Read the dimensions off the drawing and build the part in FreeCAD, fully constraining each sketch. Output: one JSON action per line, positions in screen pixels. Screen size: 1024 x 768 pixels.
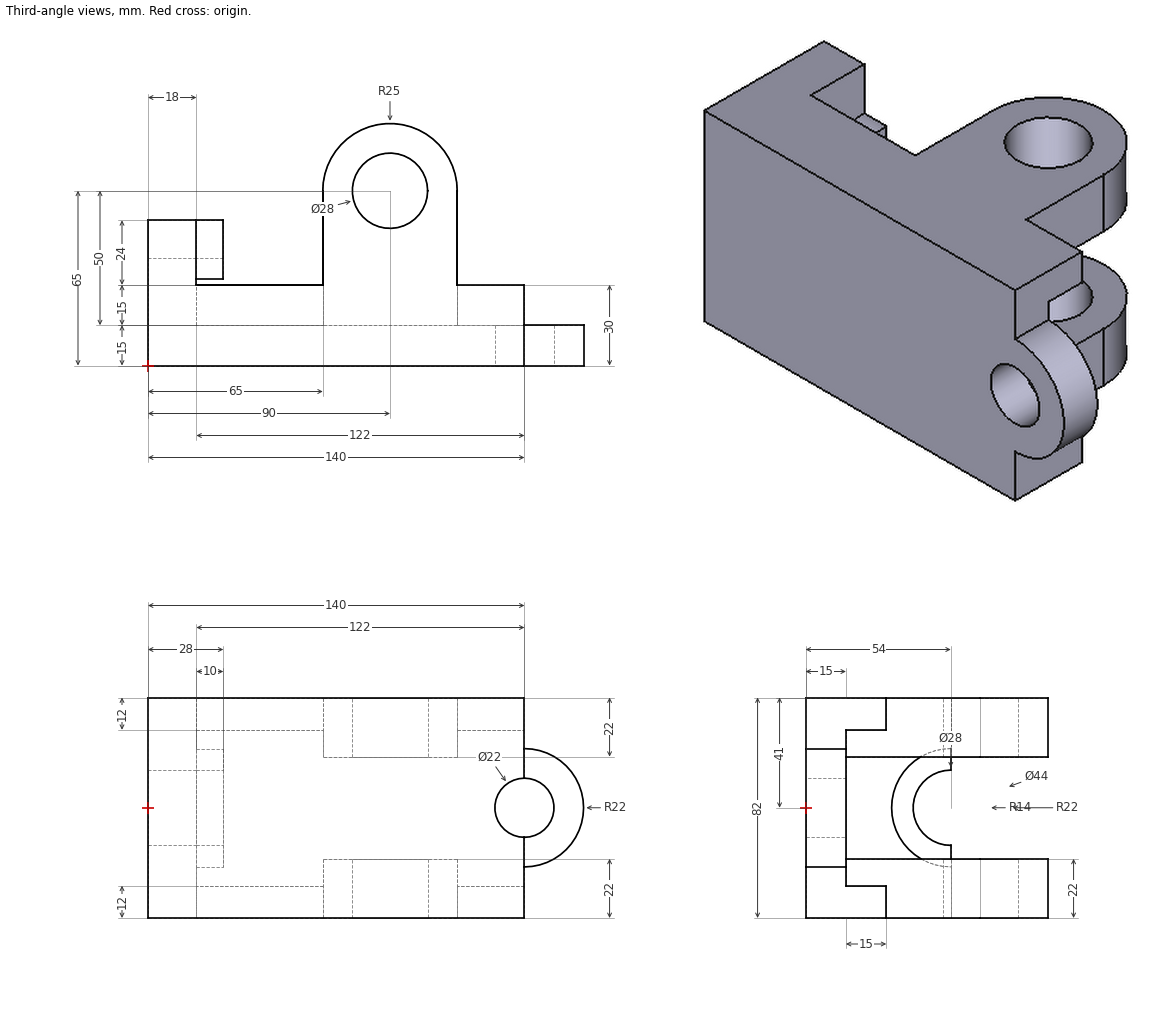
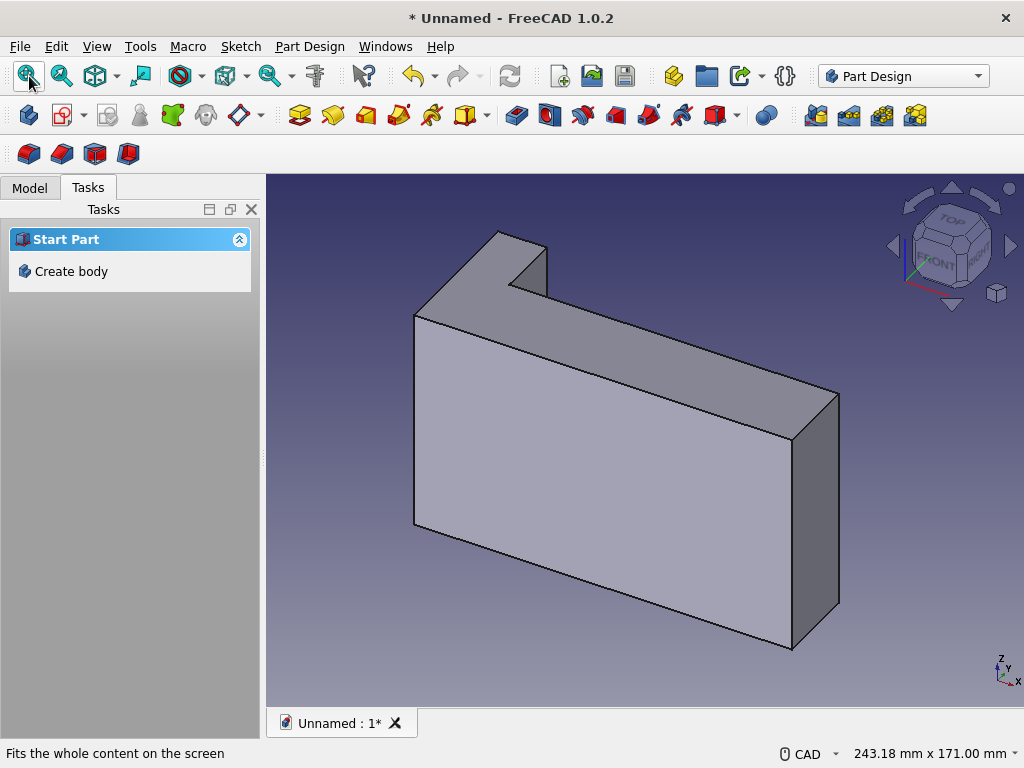
{"action": "left_click", "coordinate": [815, 461]}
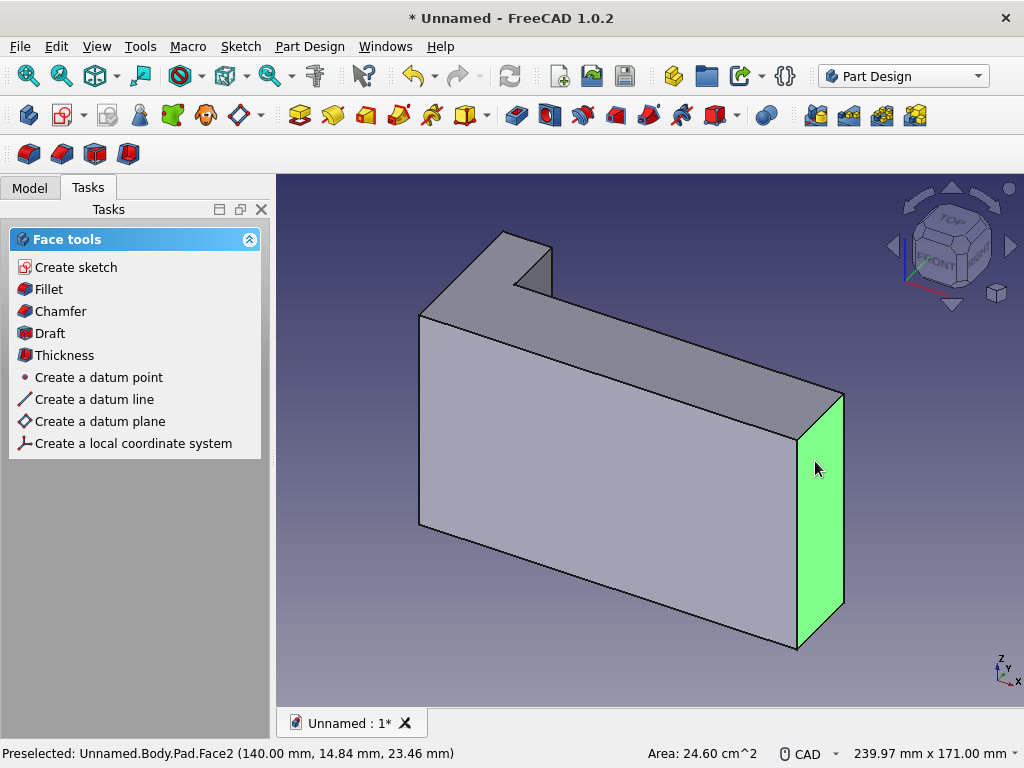
{"action": "left_click", "coordinate": [62, 116]}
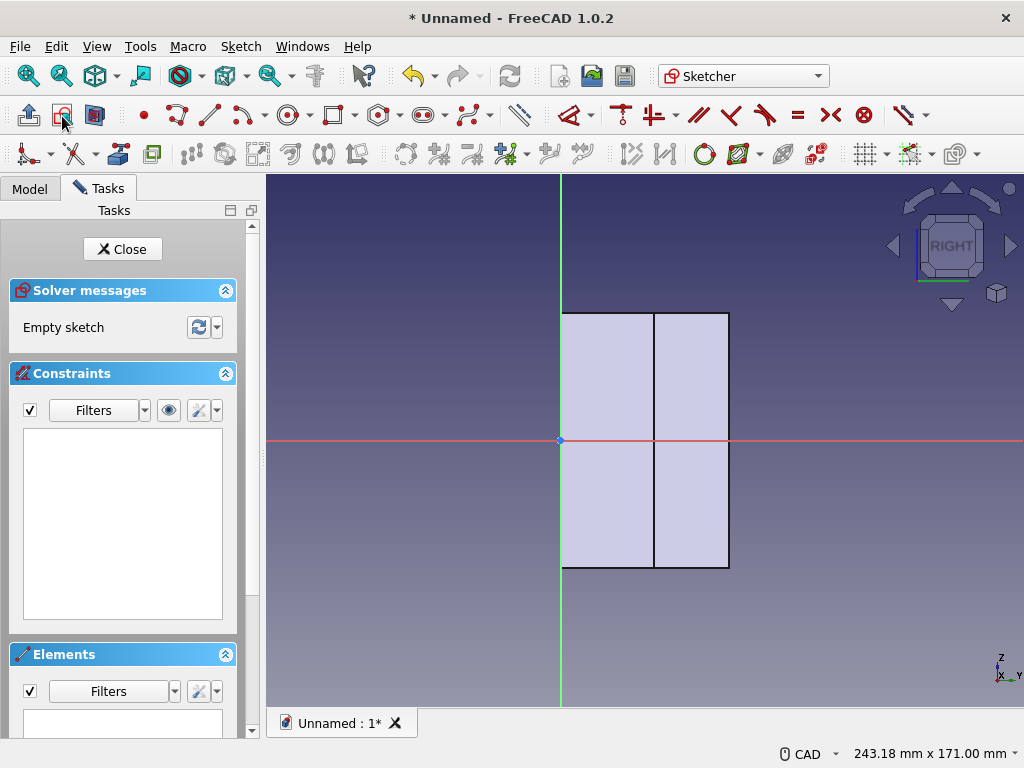
{"action": "key", "text": "g r"}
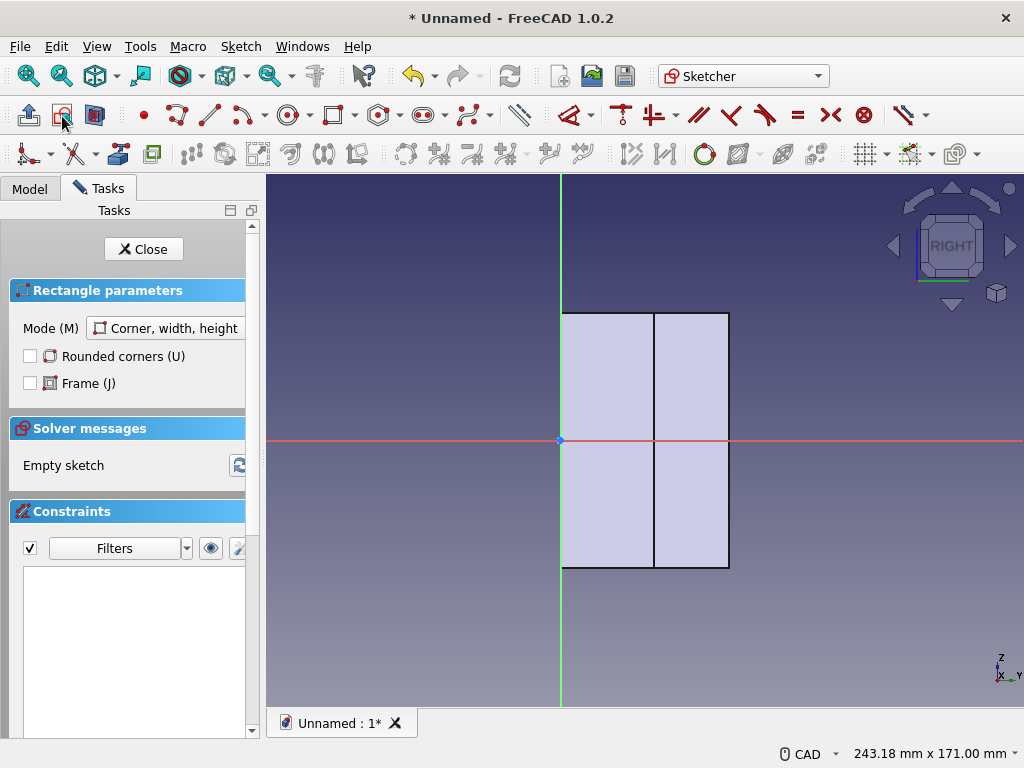
{"action": "left_click", "coordinate": [608, 313]}
{"action": "left_click", "coordinate": [654, 568]}
{"action": "key", "text": "Escape"}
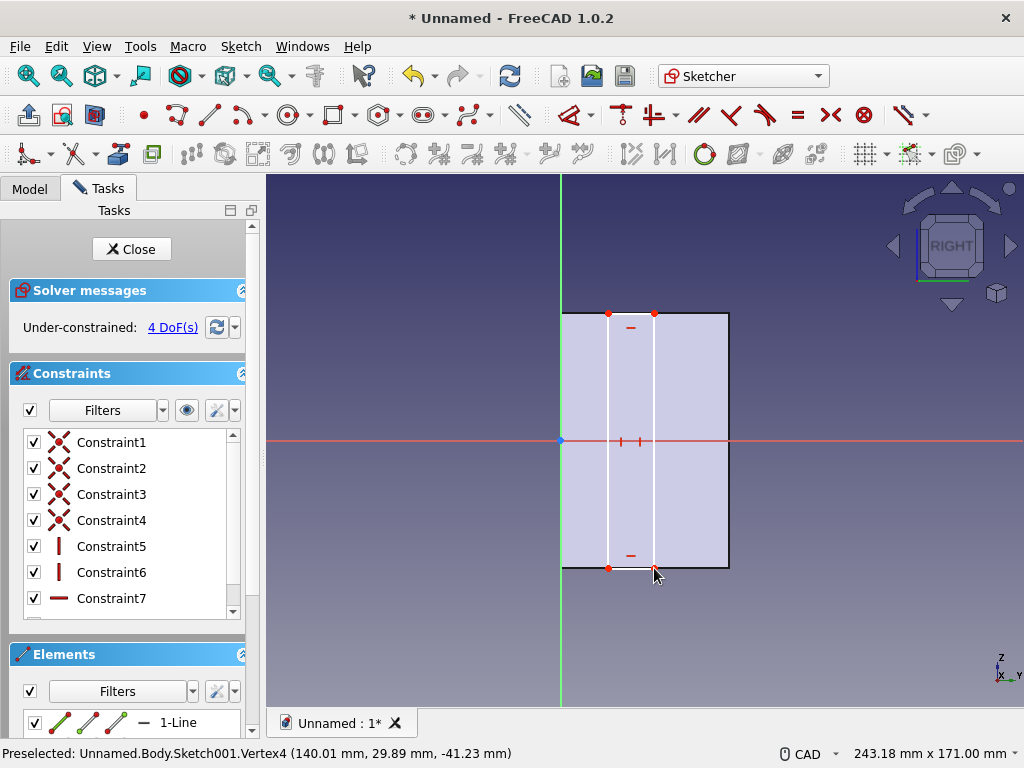
{"action": "key", "text": "d"}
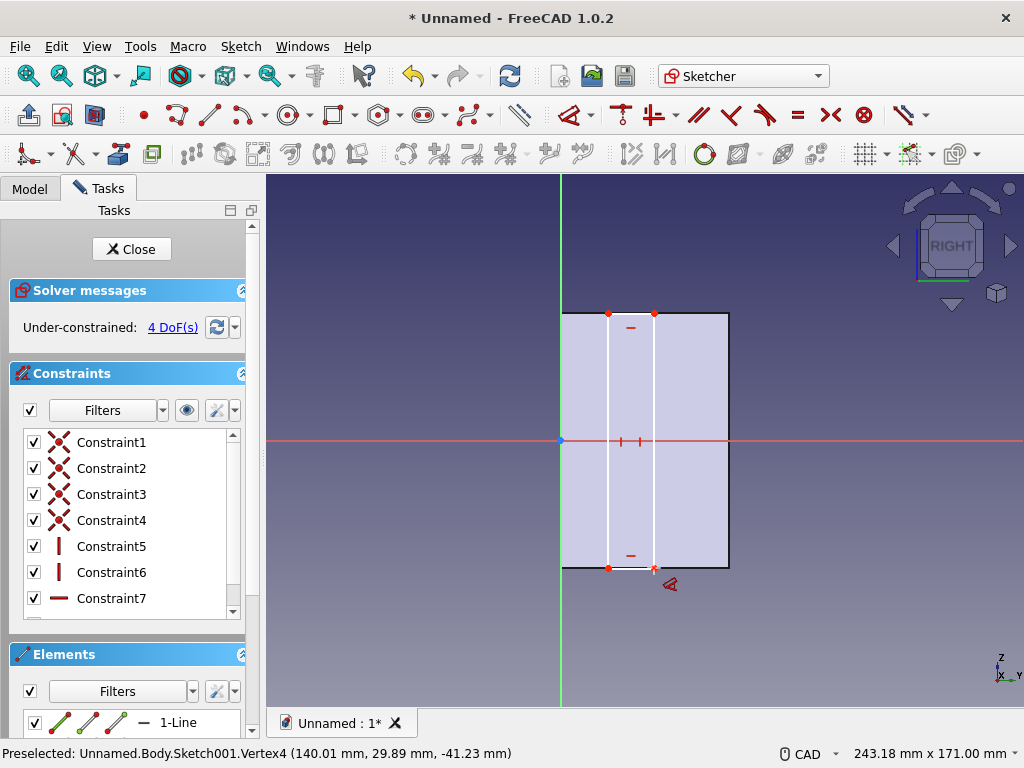
{"action": "left_click", "coordinate": [608, 390]}
{"action": "left_click", "coordinate": [574, 383]}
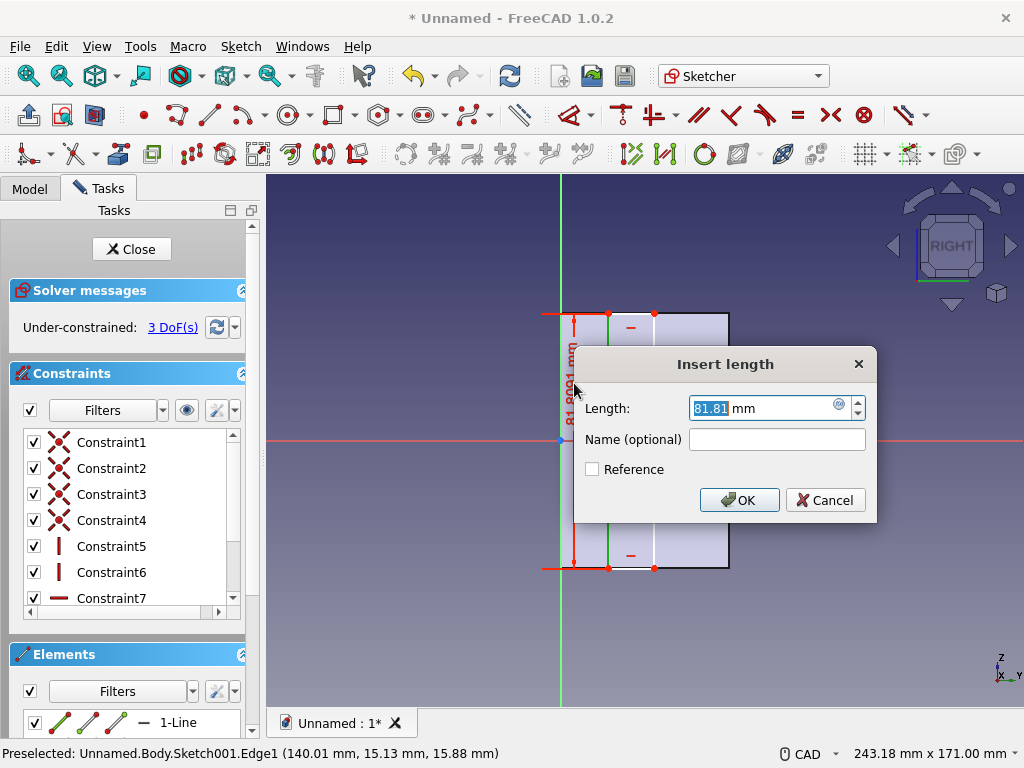
{"action": "type", "text": "82"}
{"action": "key", "text": "Return"}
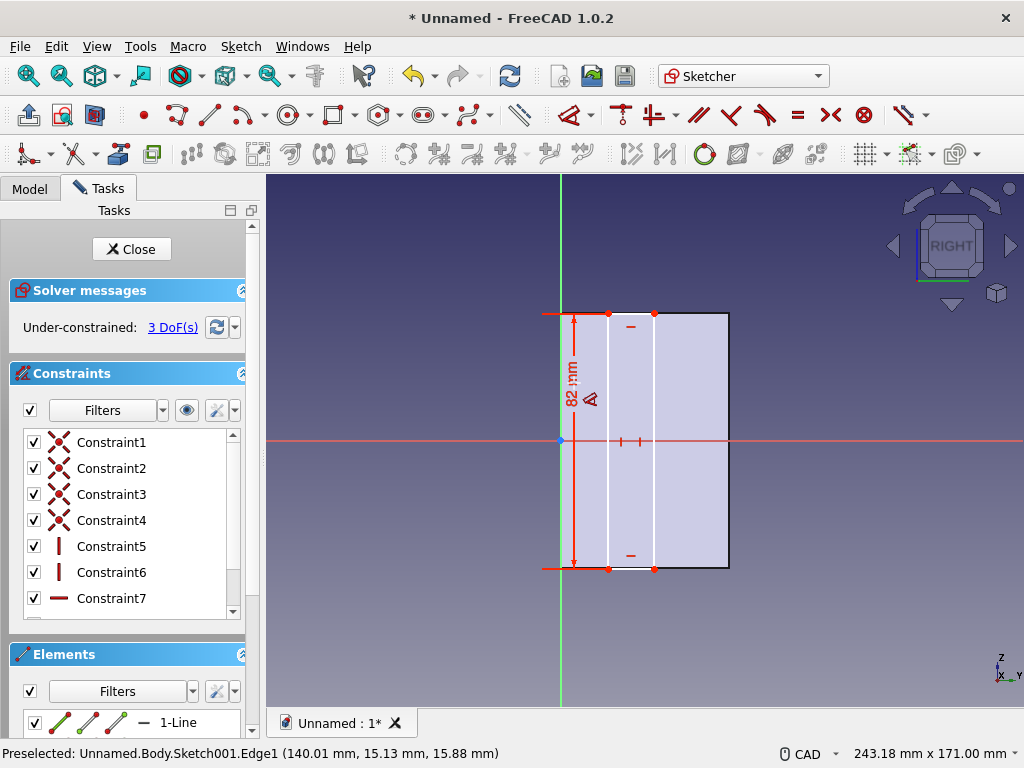
{"action": "left_click", "coordinate": [622, 569]}
{"action": "left_click", "coordinate": [631, 603]}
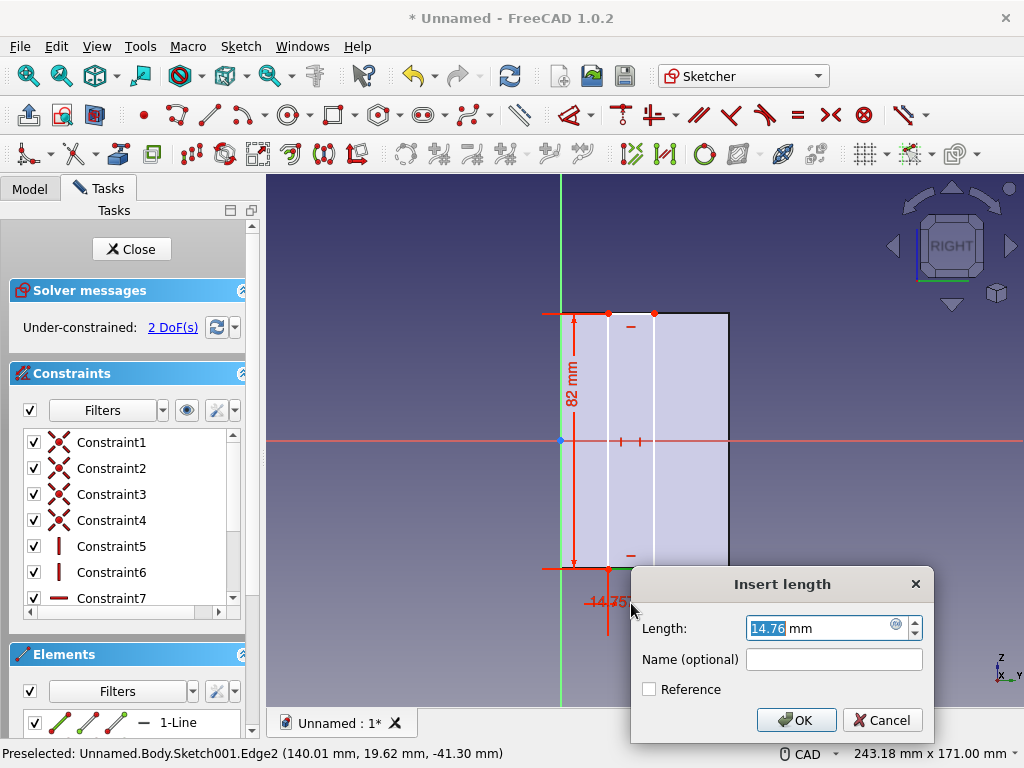
{"action": "type", "text": "15"}
{"action": "key", "text": "Return"}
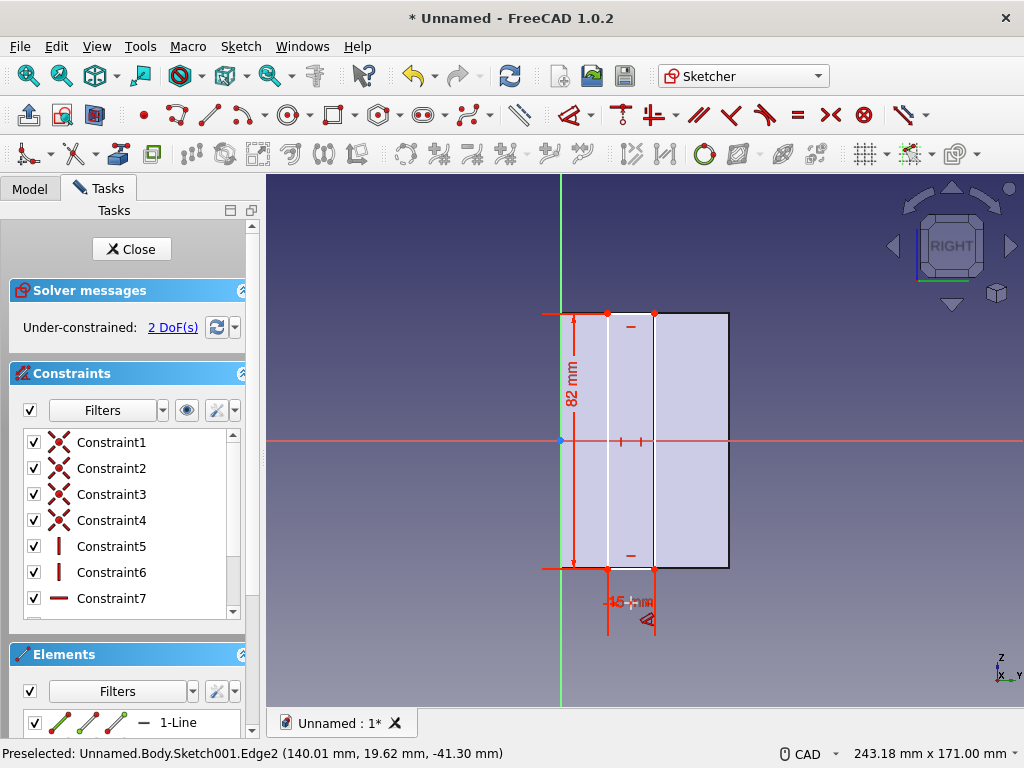
{"action": "left_click", "coordinate": [608, 314]}
{"action": "left_click", "coordinate": [584, 280]}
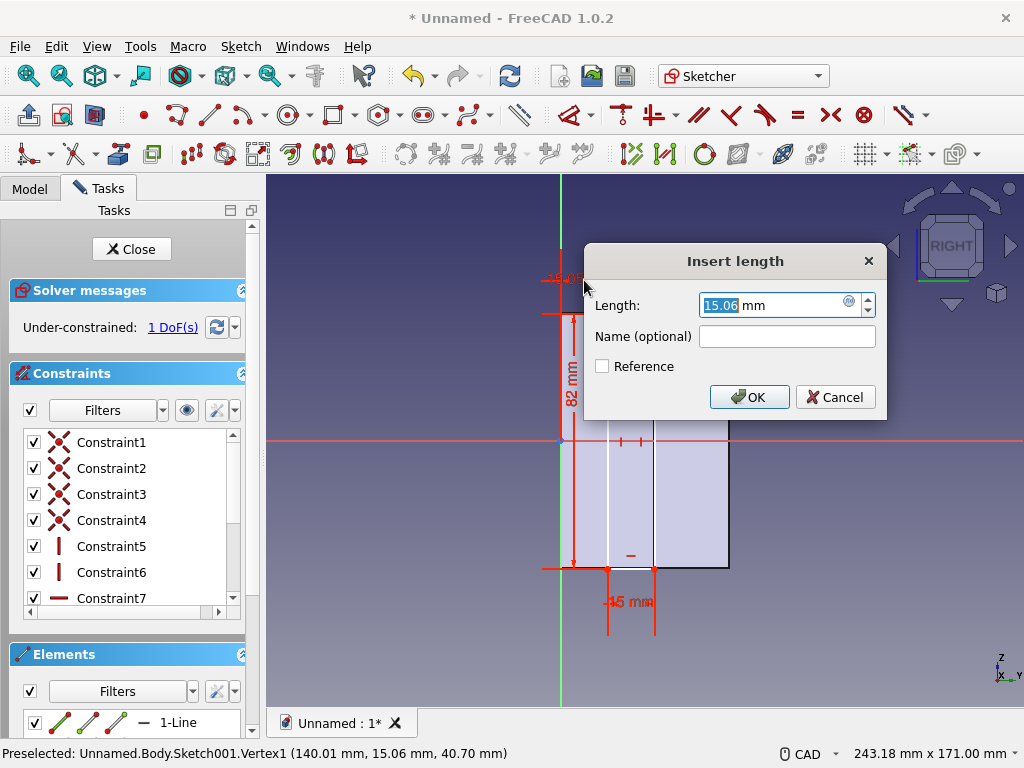
{"action": "type", "text": "15"}
{"action": "key", "text": "Return"}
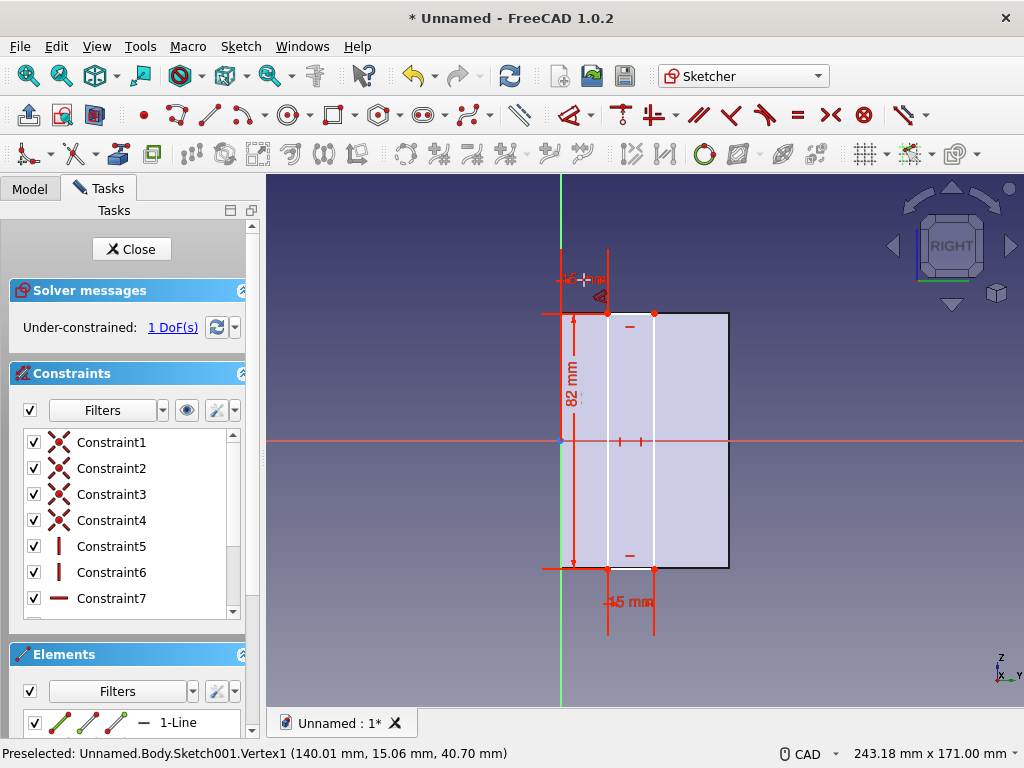
{"action": "left_click", "coordinate": [608, 314]}
{"action": "left_click", "coordinate": [527, 348]}